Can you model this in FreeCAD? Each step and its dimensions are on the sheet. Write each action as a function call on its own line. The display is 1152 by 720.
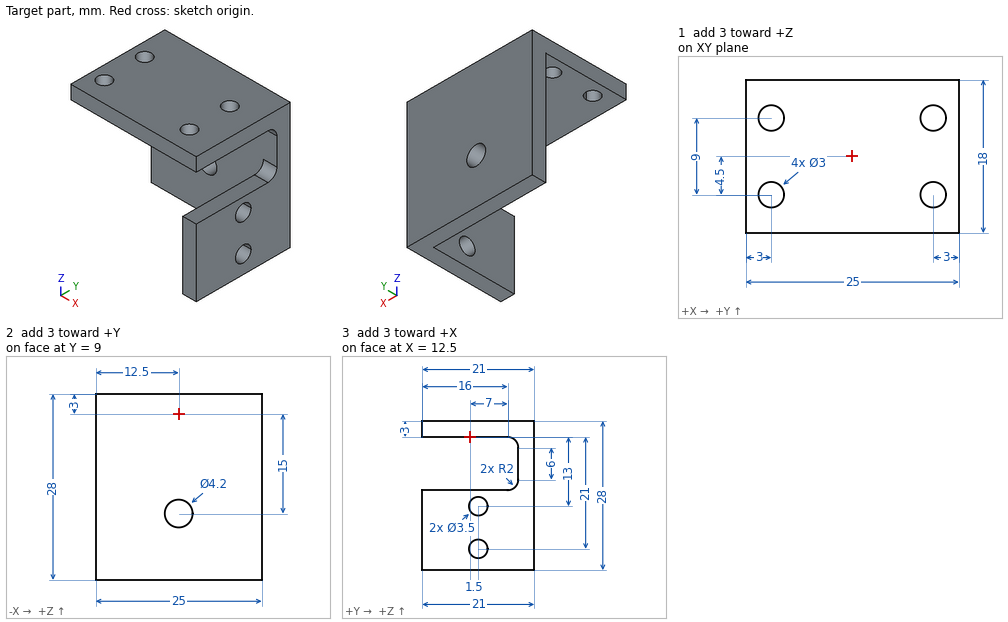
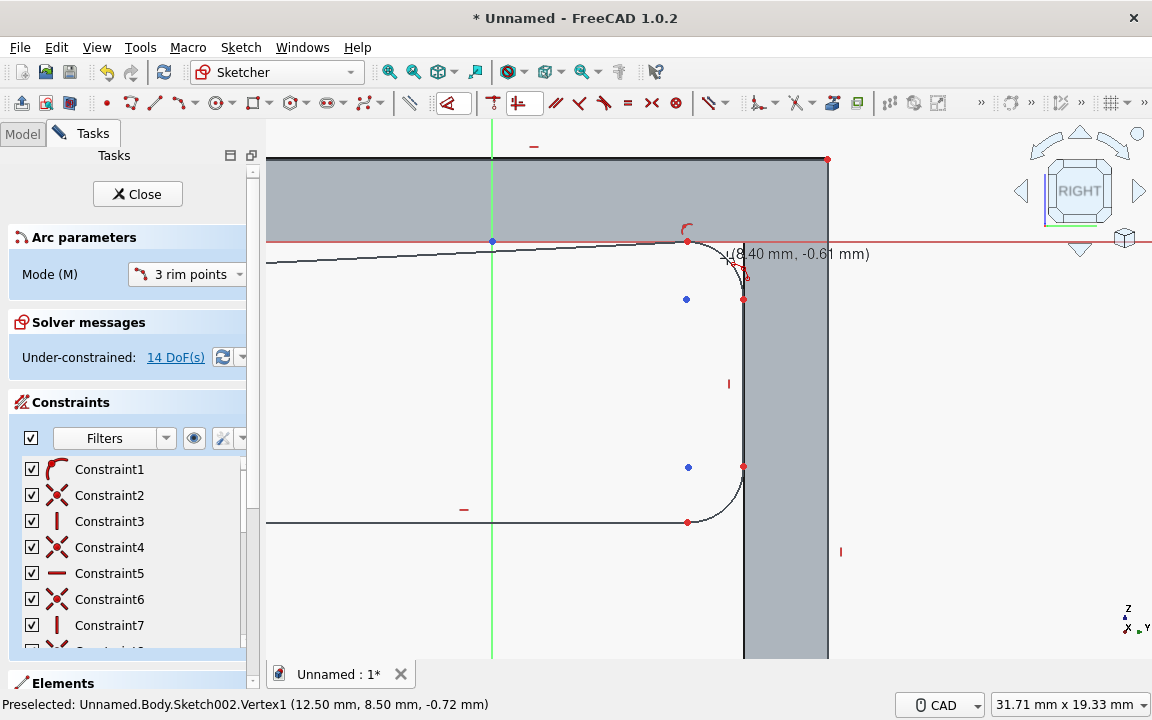
click(216, 104)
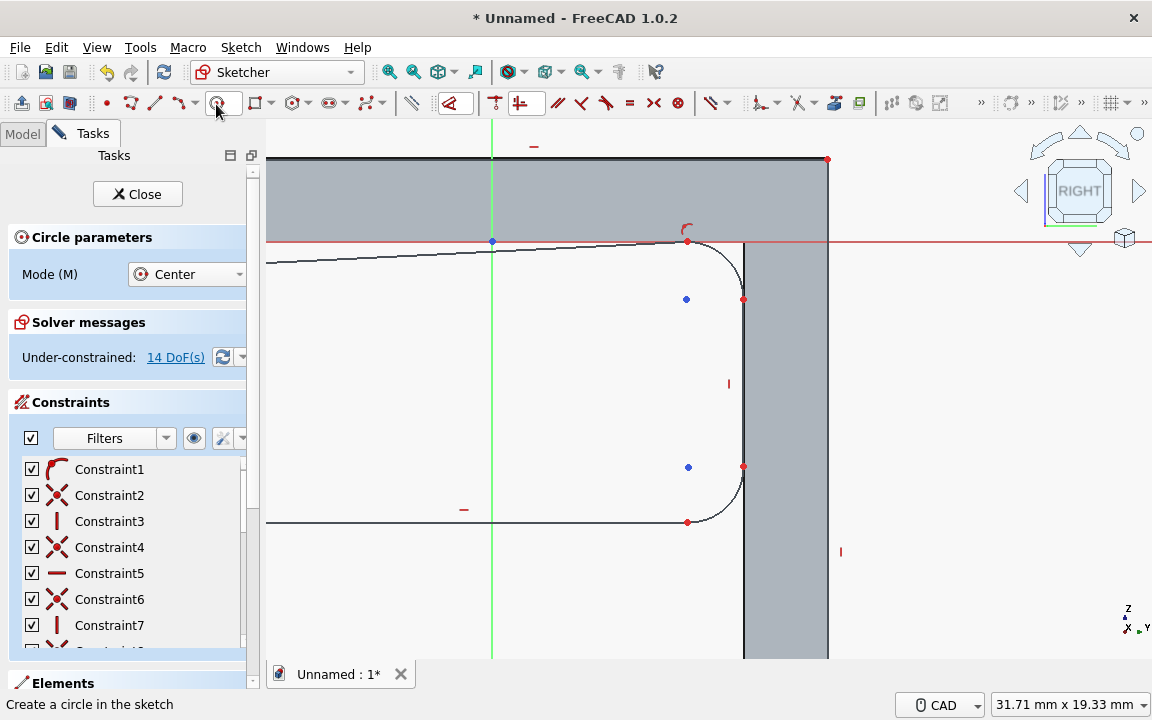
click(534, 605)
click(569, 571)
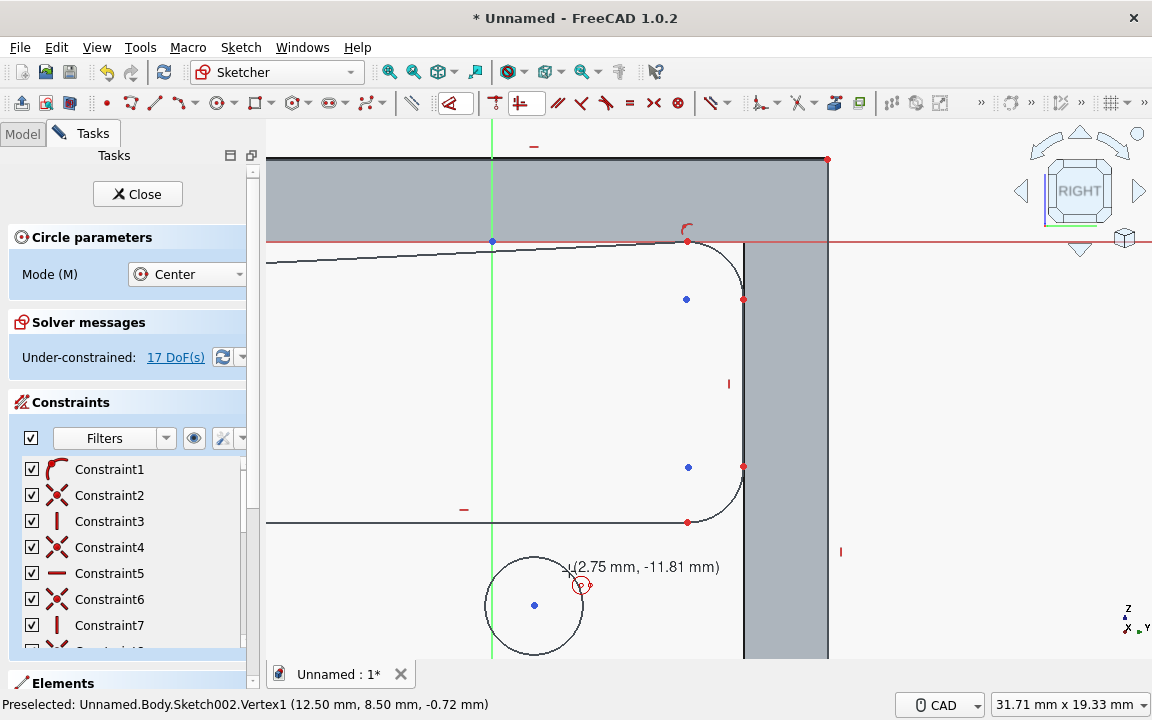
scroll(727, 258, down, 4)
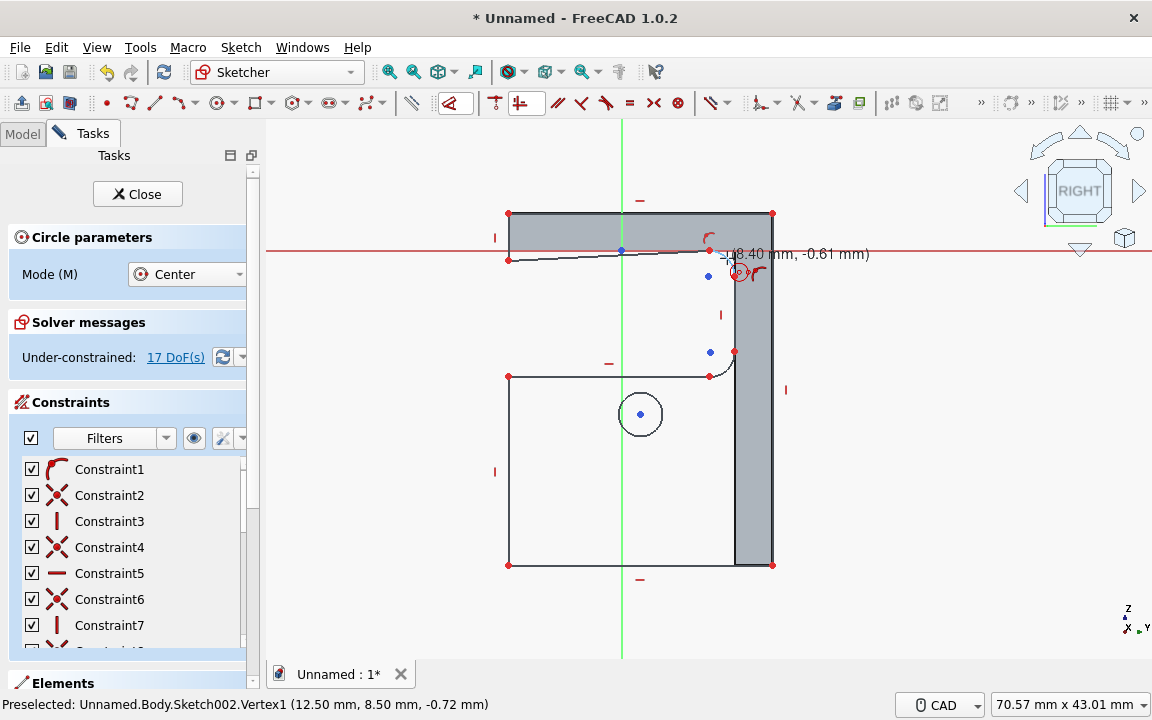
click(641, 515)
click(656, 499)
key(Escape)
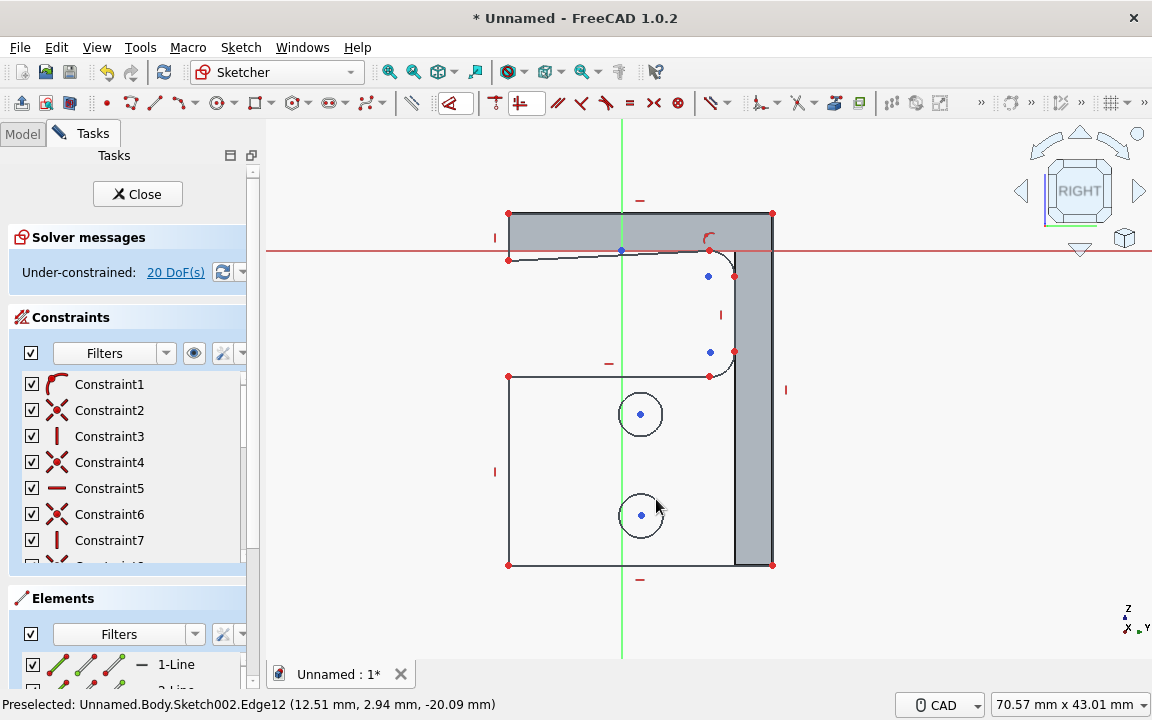
click(649, 254)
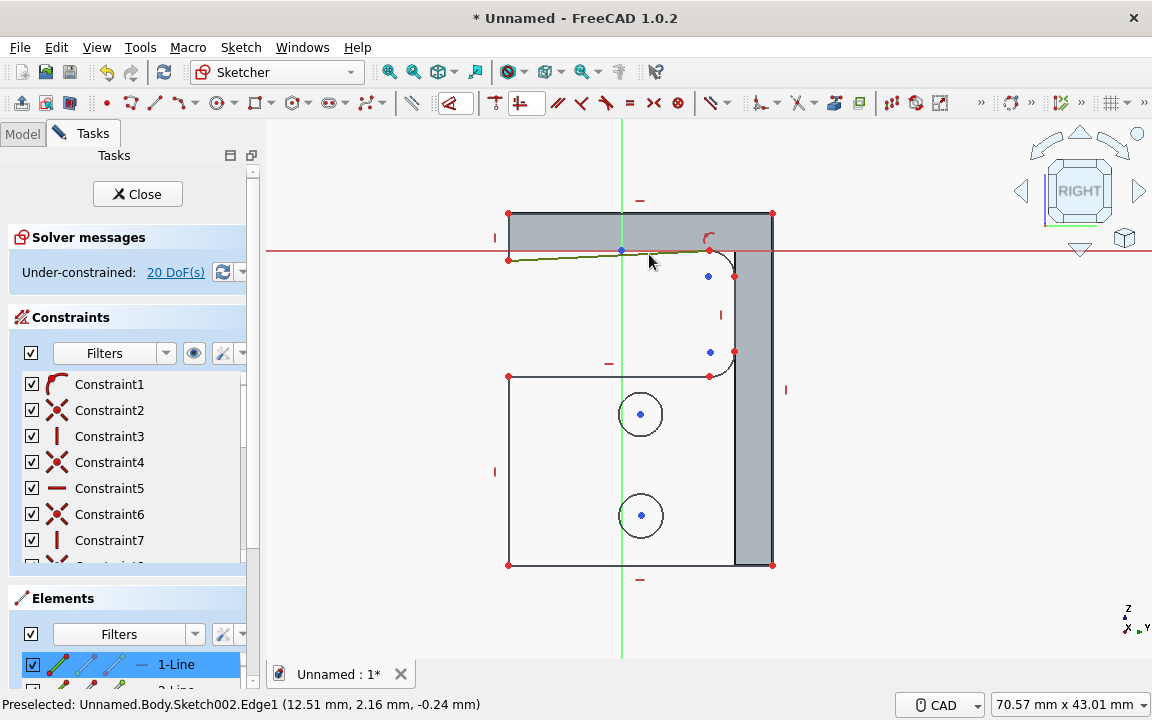
click(732, 265)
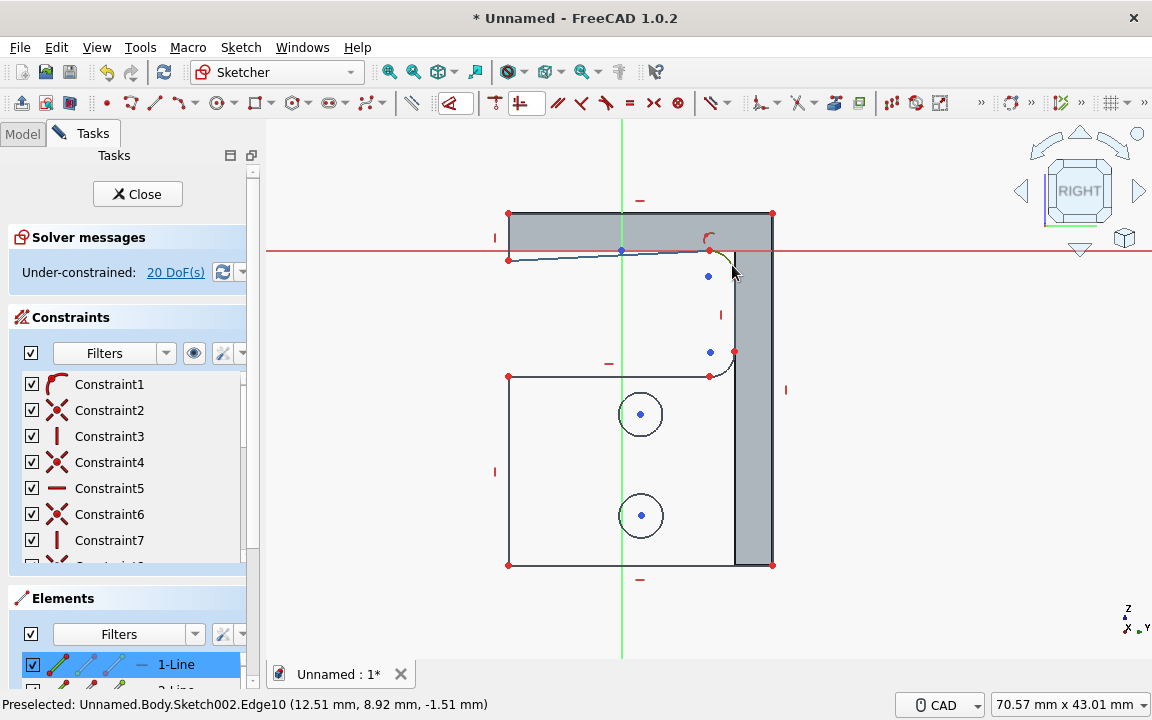
key(t)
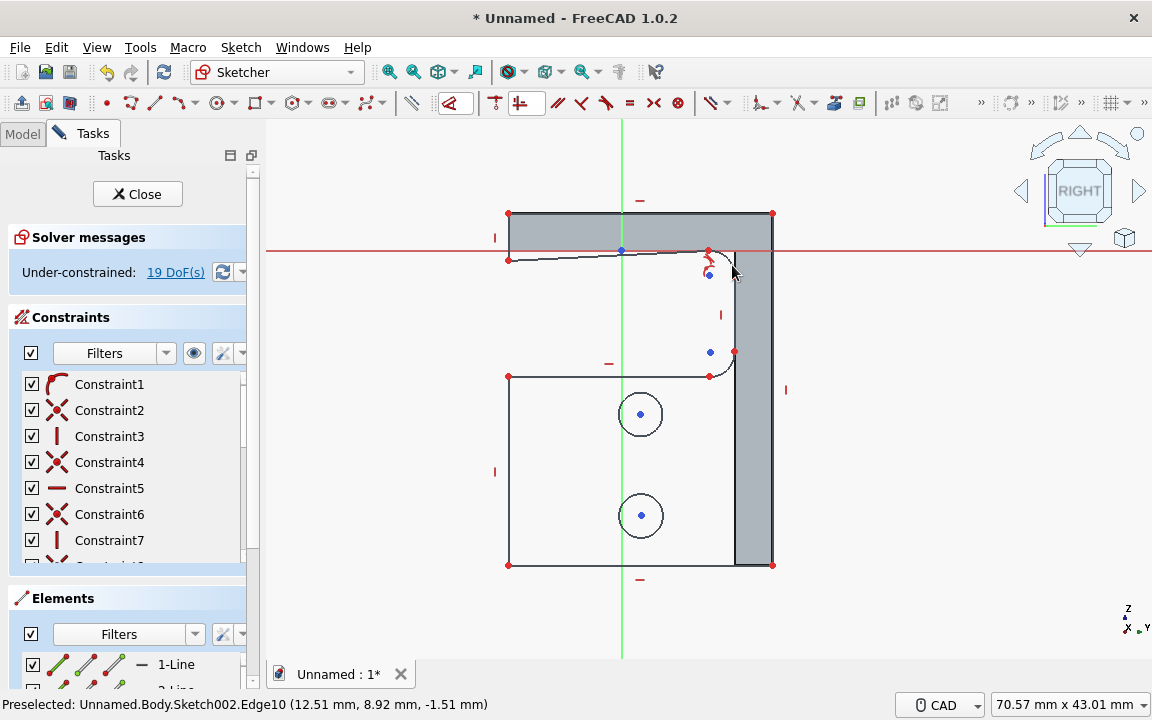
click(569, 377)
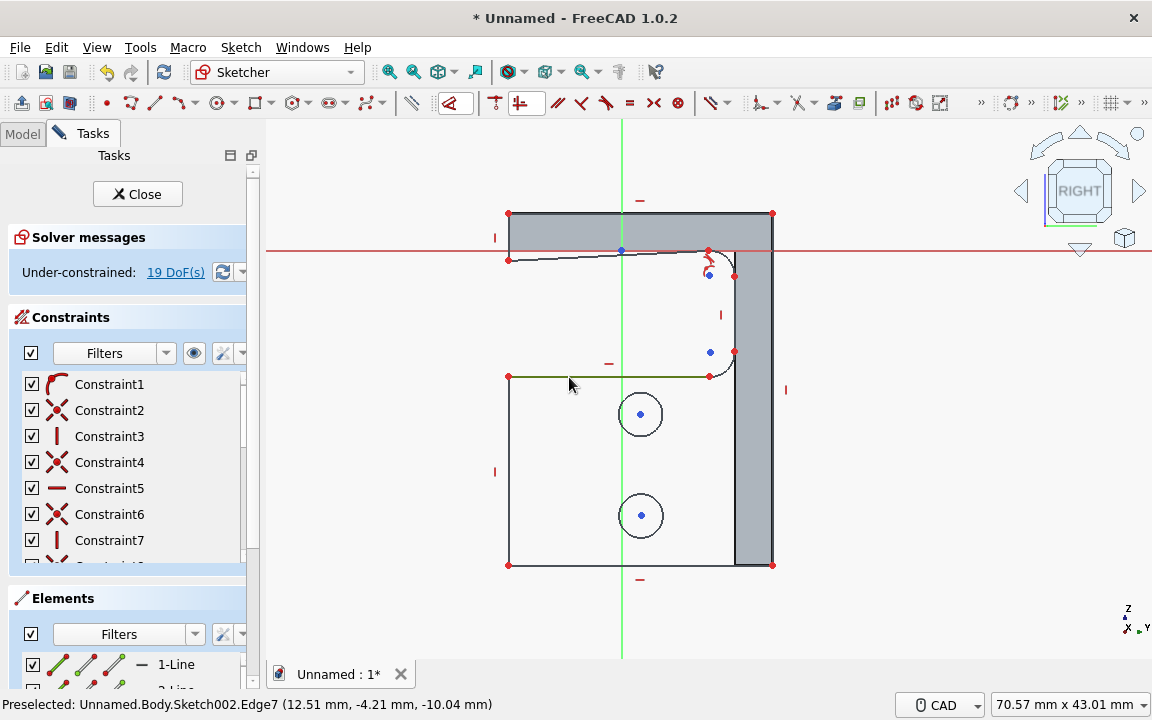
click(721, 374)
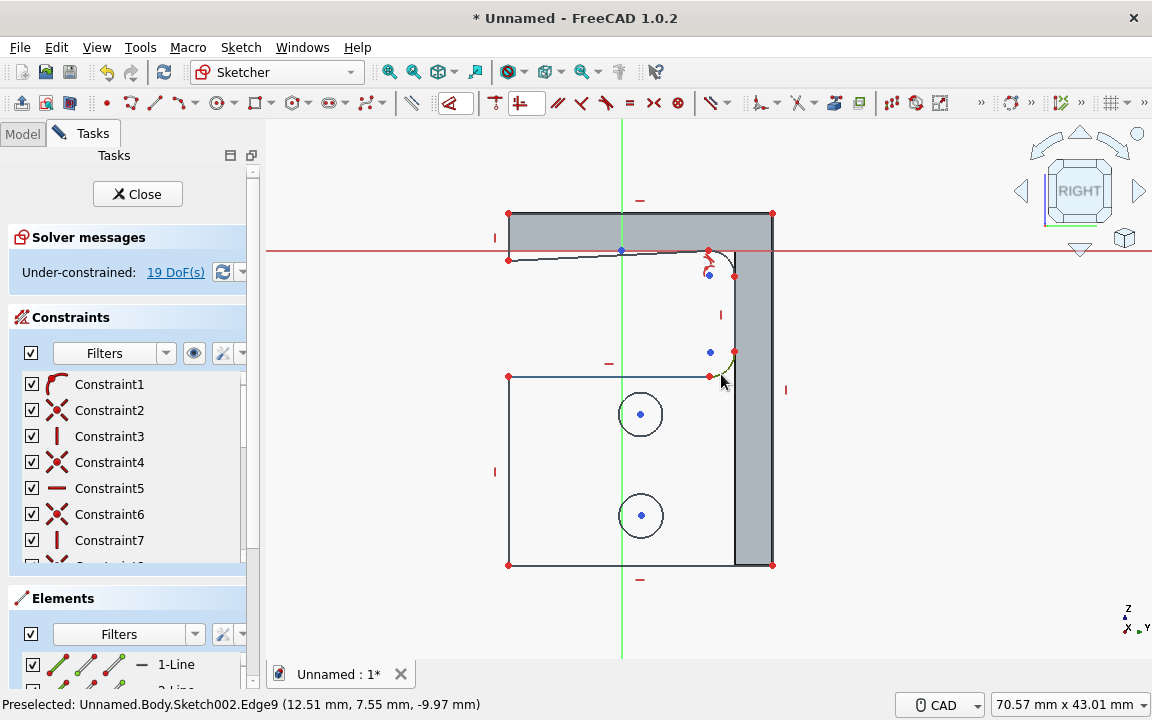
click(606, 104)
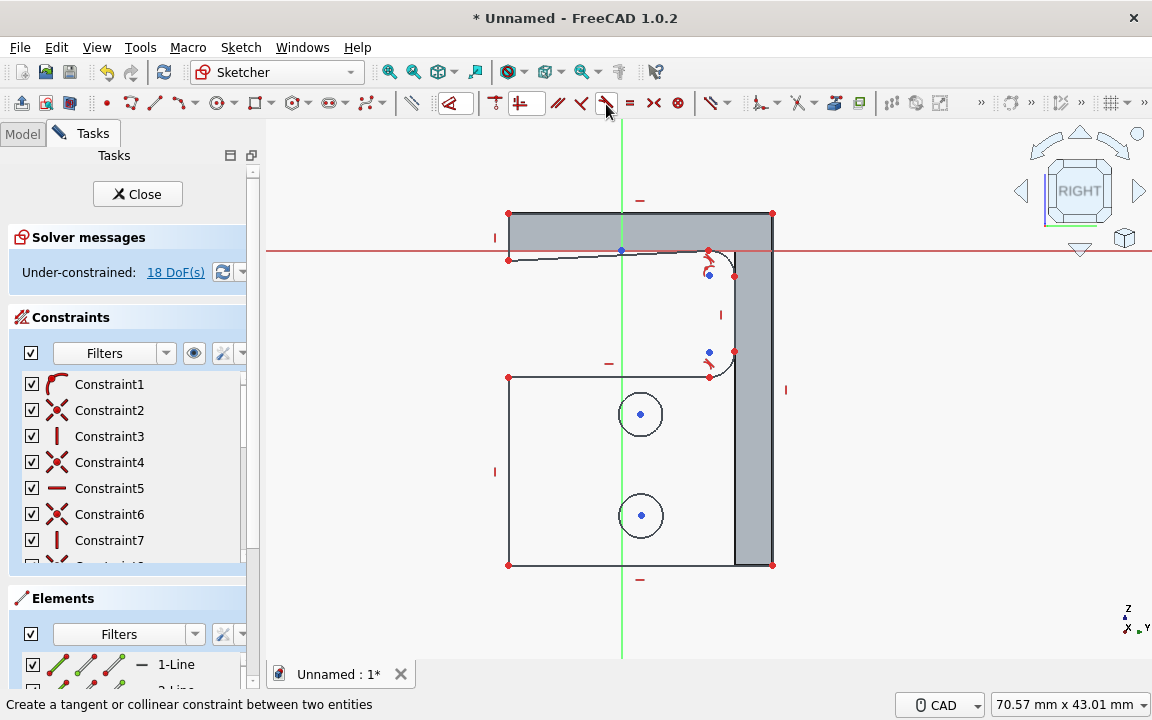
click(735, 330)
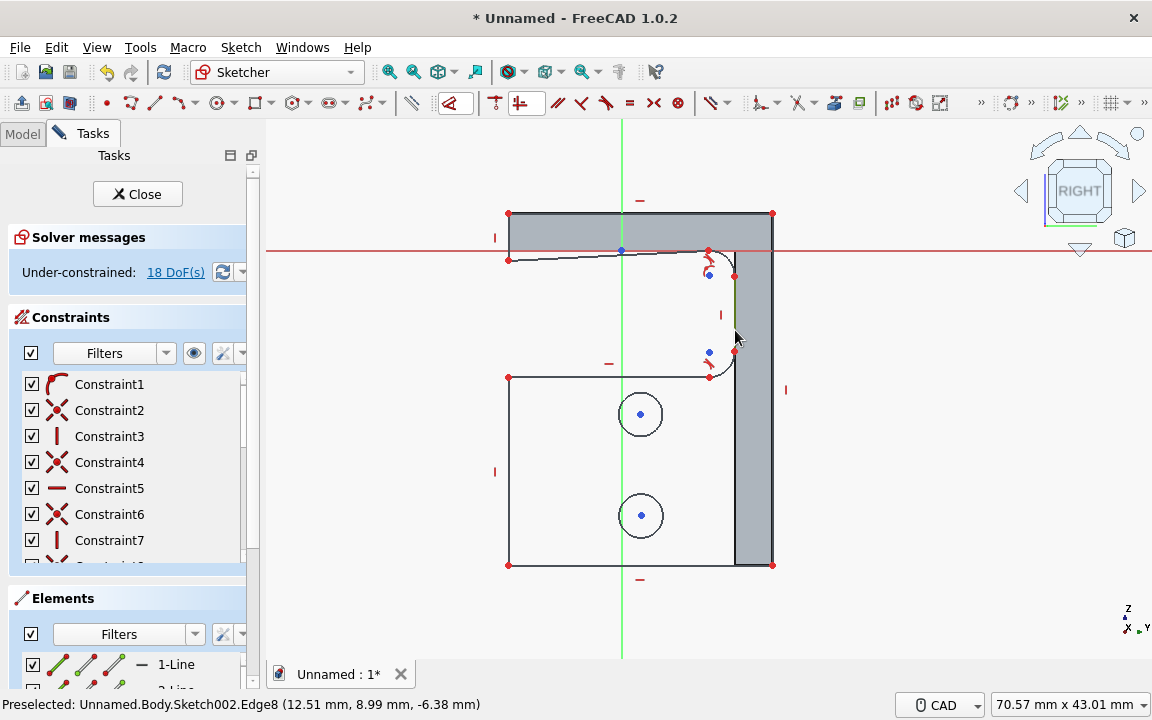
click(721, 374)